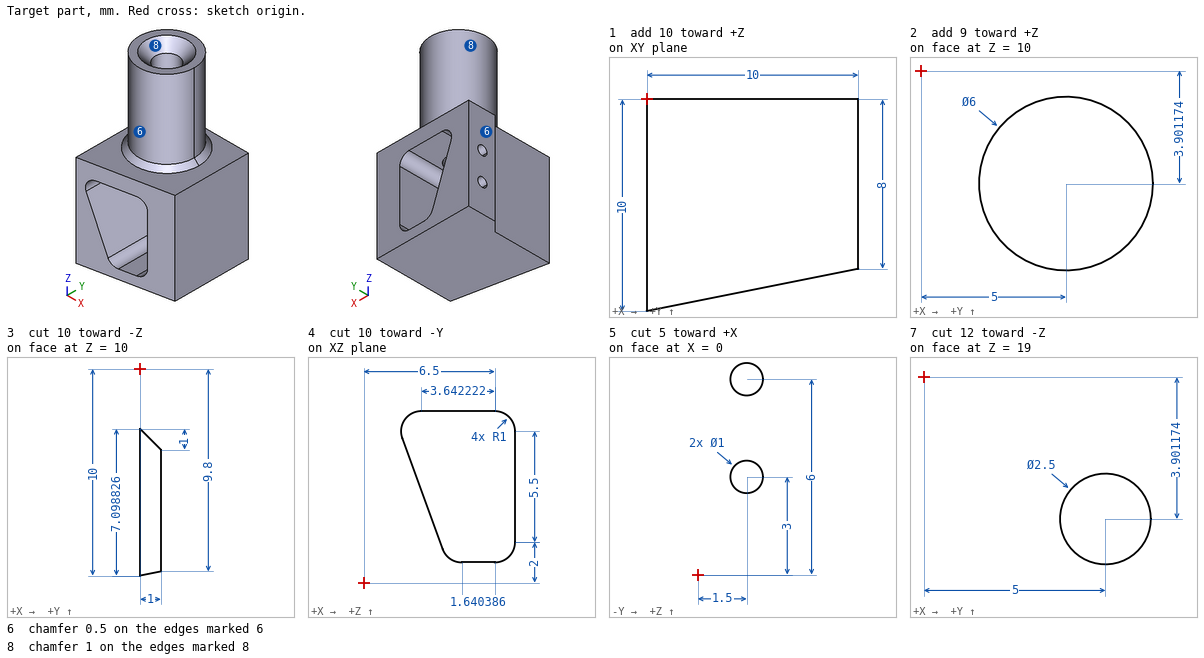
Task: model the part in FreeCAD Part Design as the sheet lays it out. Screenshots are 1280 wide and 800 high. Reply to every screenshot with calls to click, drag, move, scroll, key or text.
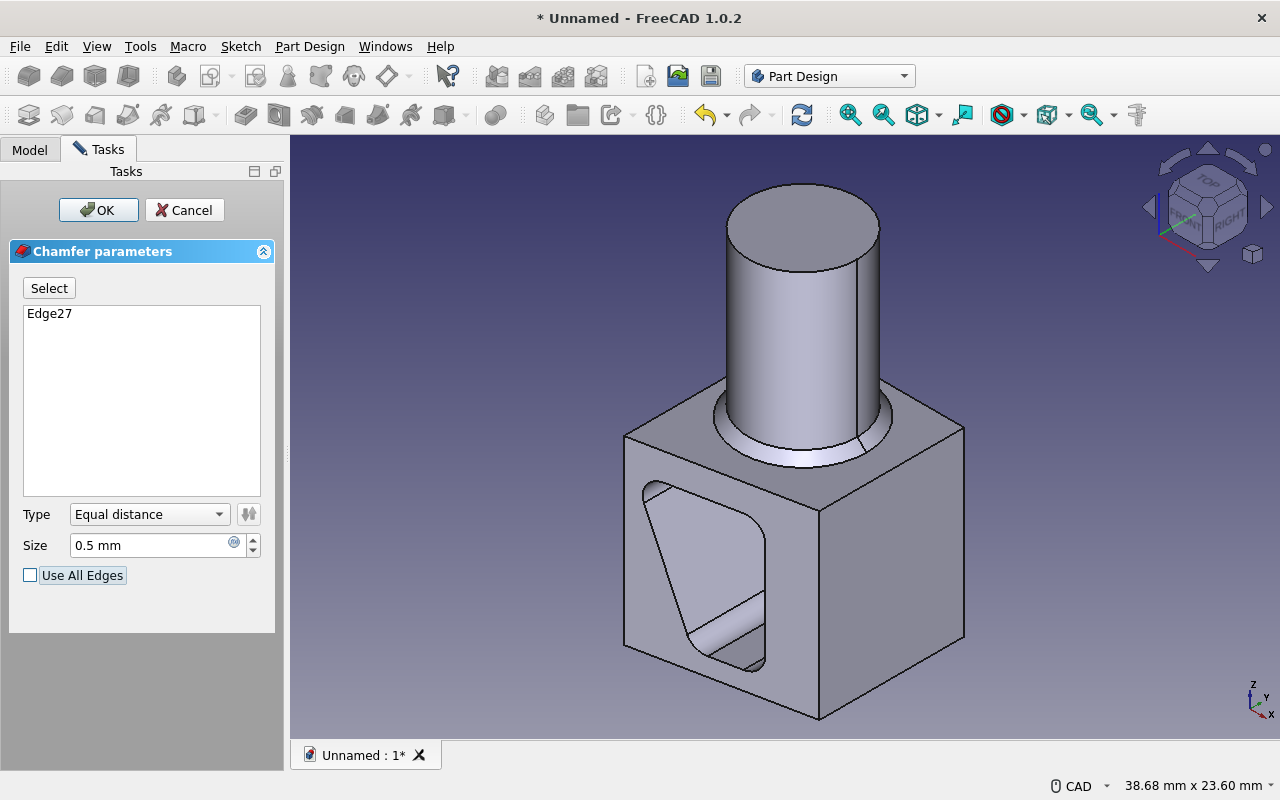
click(99, 210)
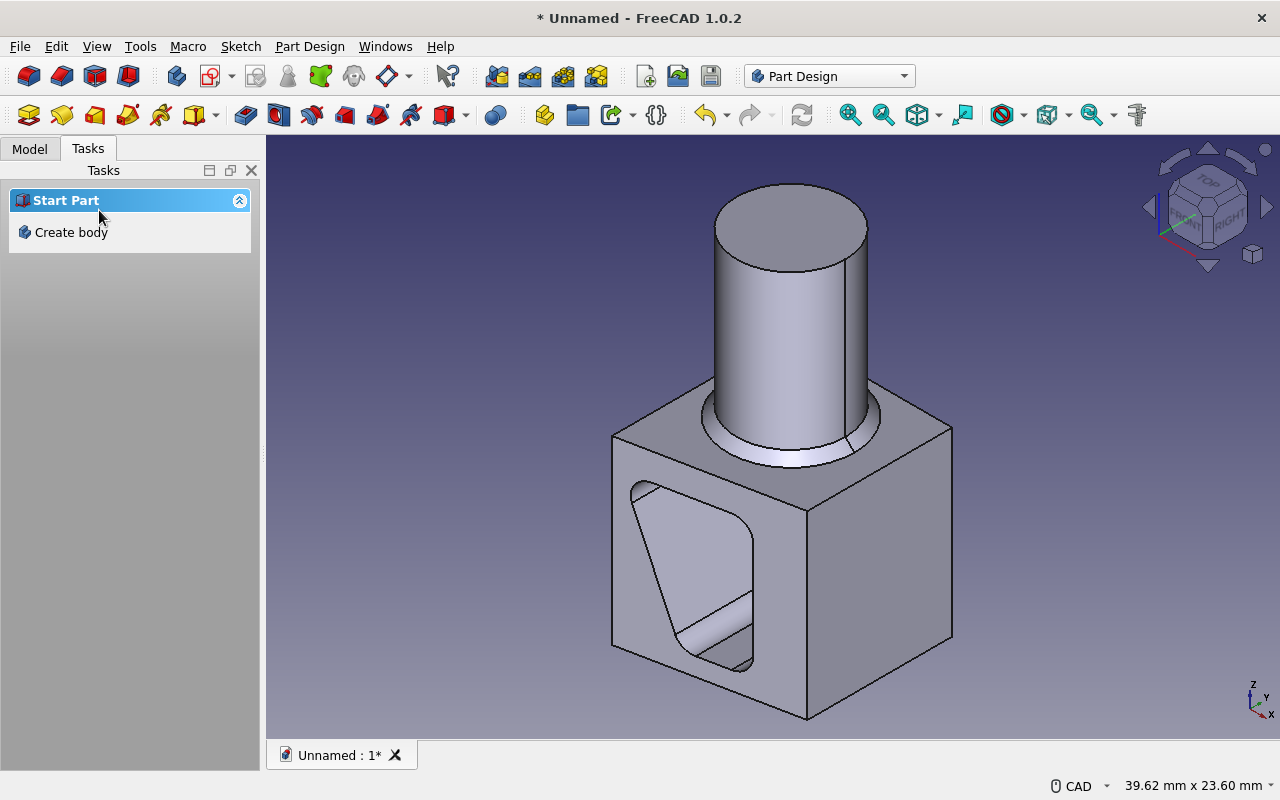
click(851, 116)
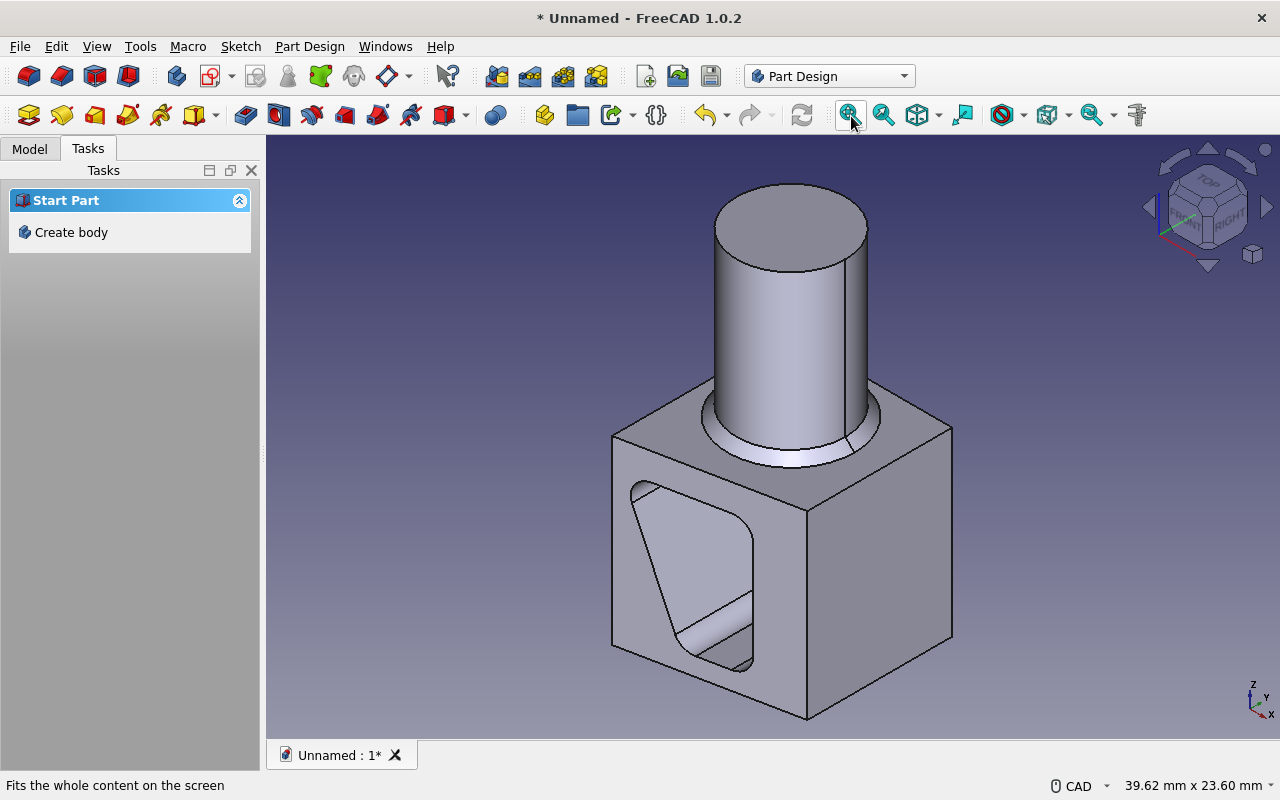
click(791, 227)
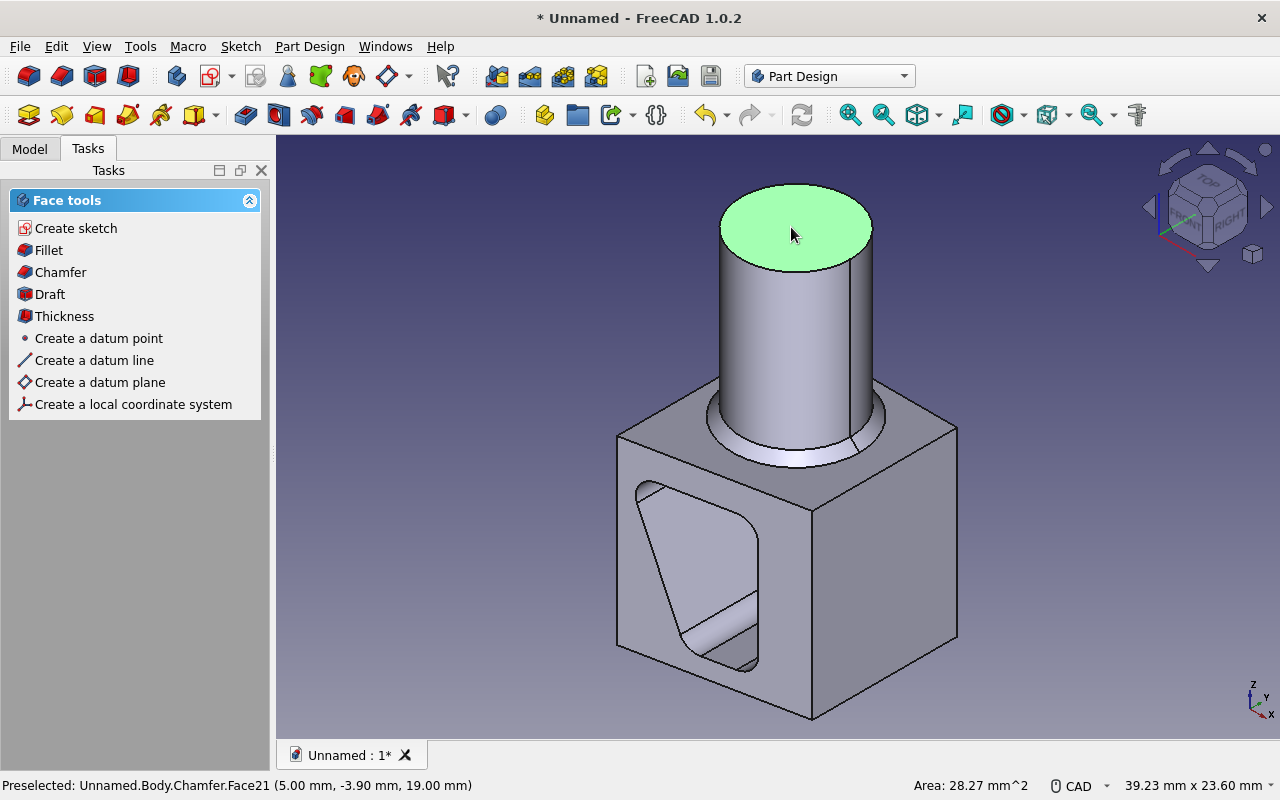
click(210, 76)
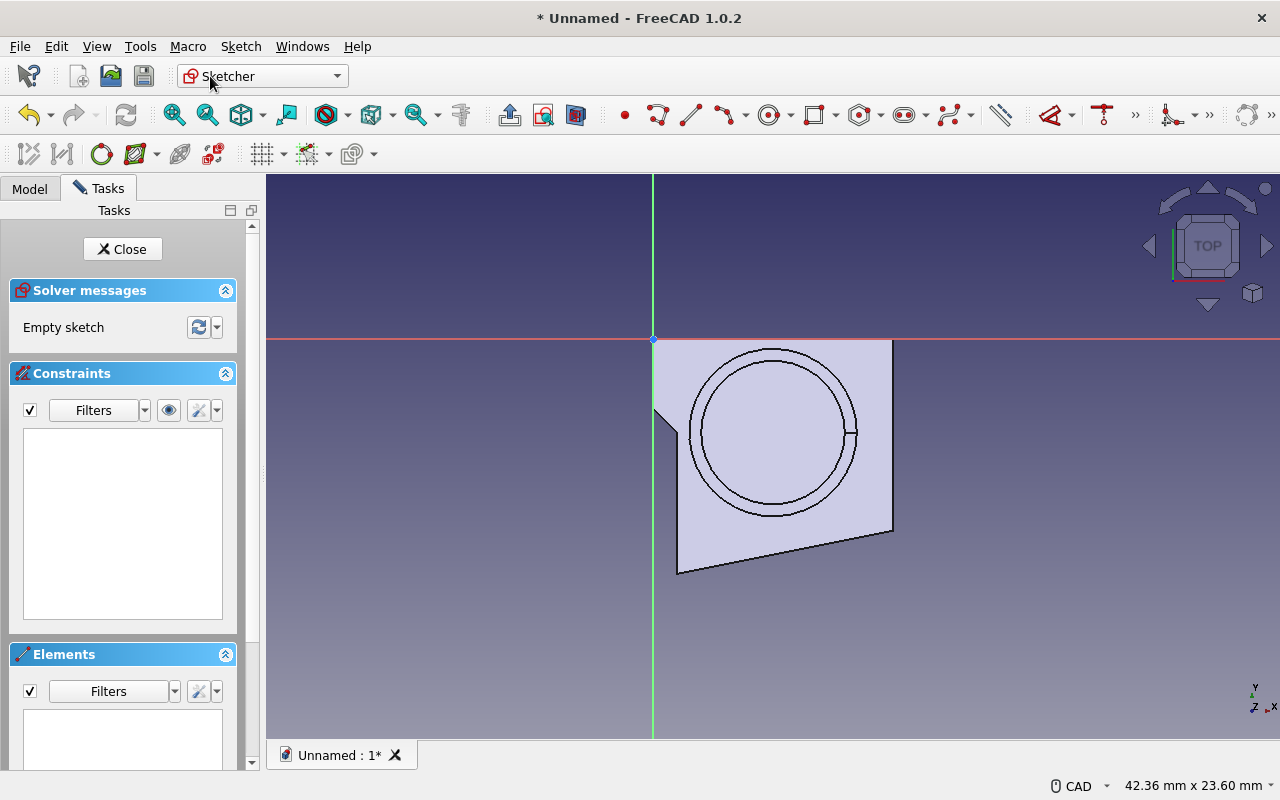
scroll(742, 368, up, 5)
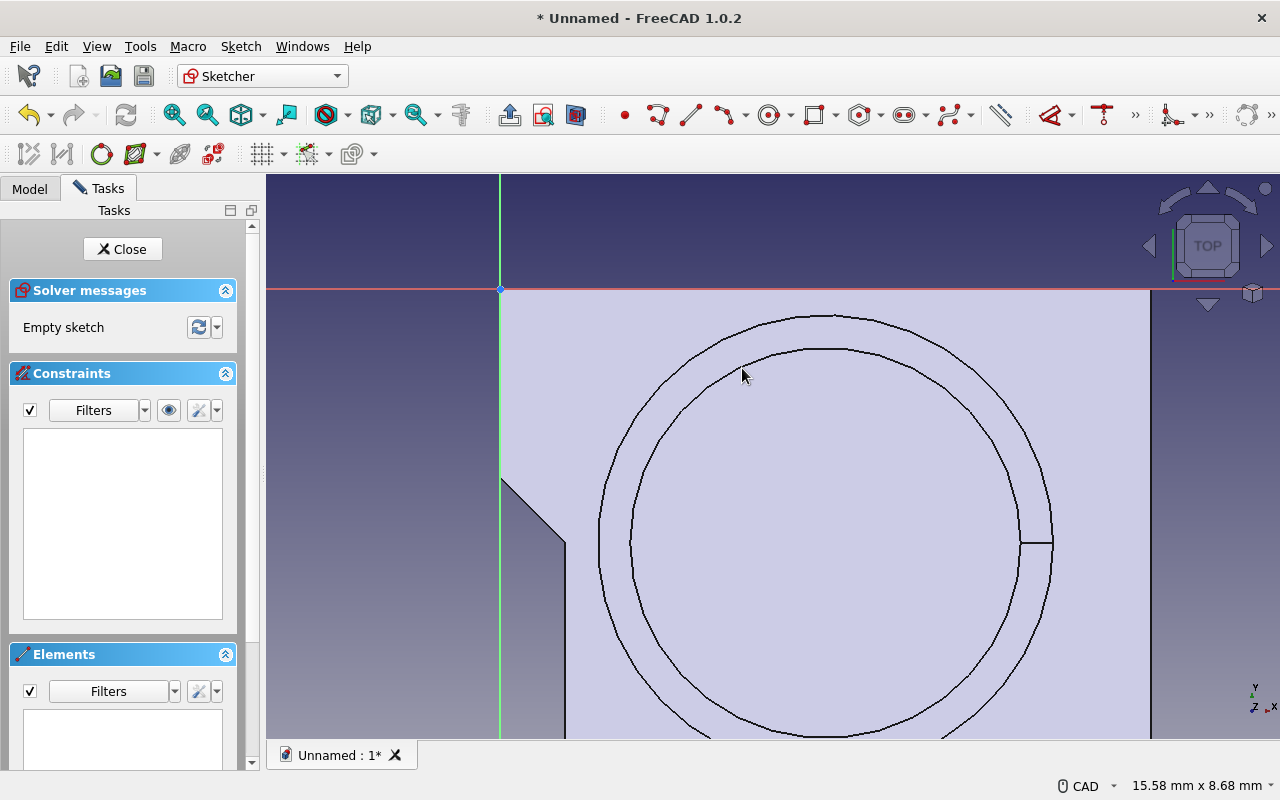
key(g)
key(c)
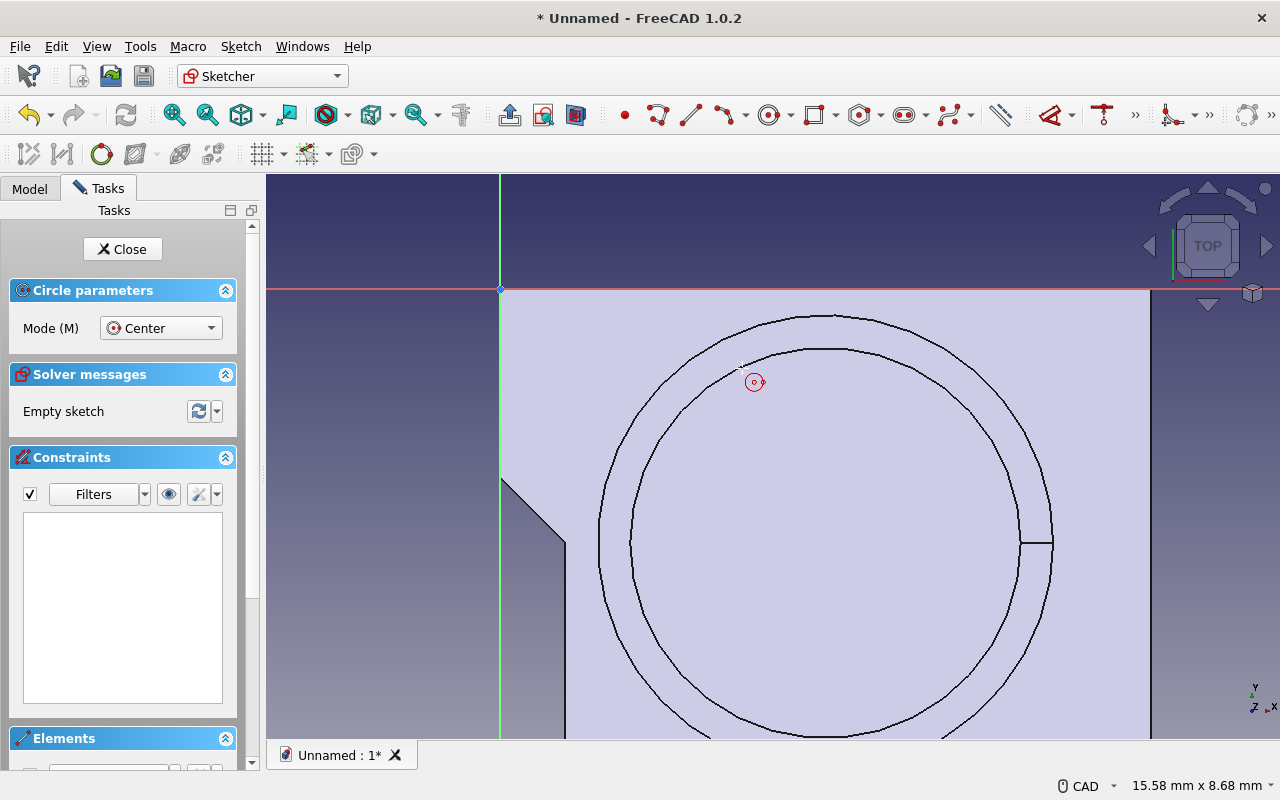
click(825, 543)
click(883, 485)
key(Escape)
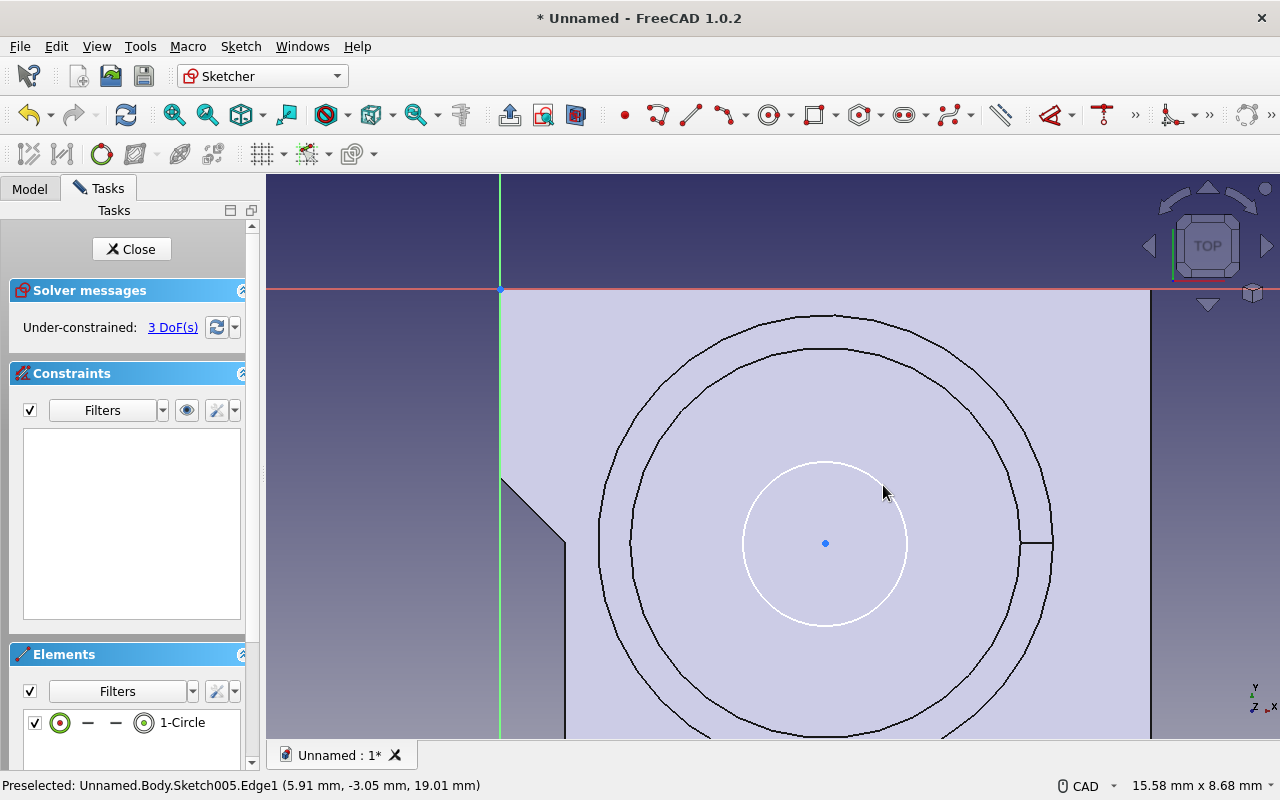
key(d)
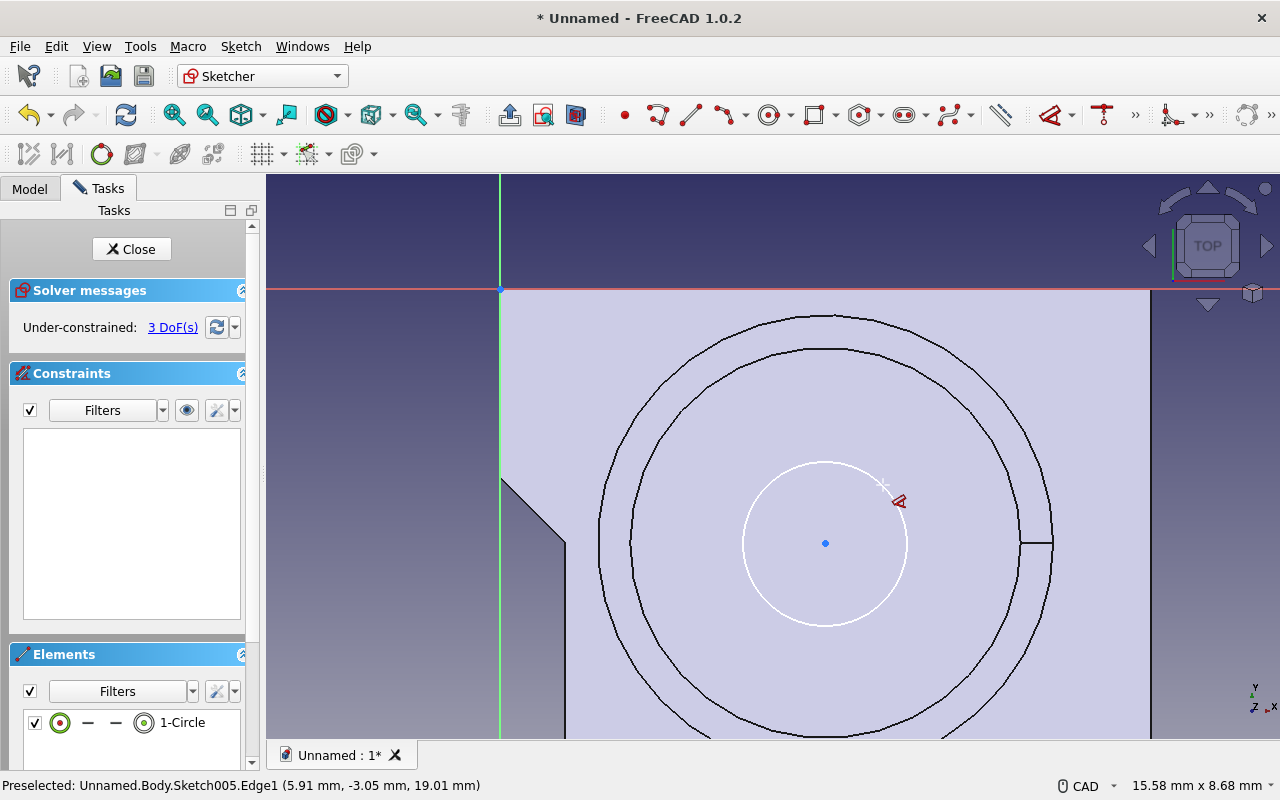
click(883, 486)
click(906, 463)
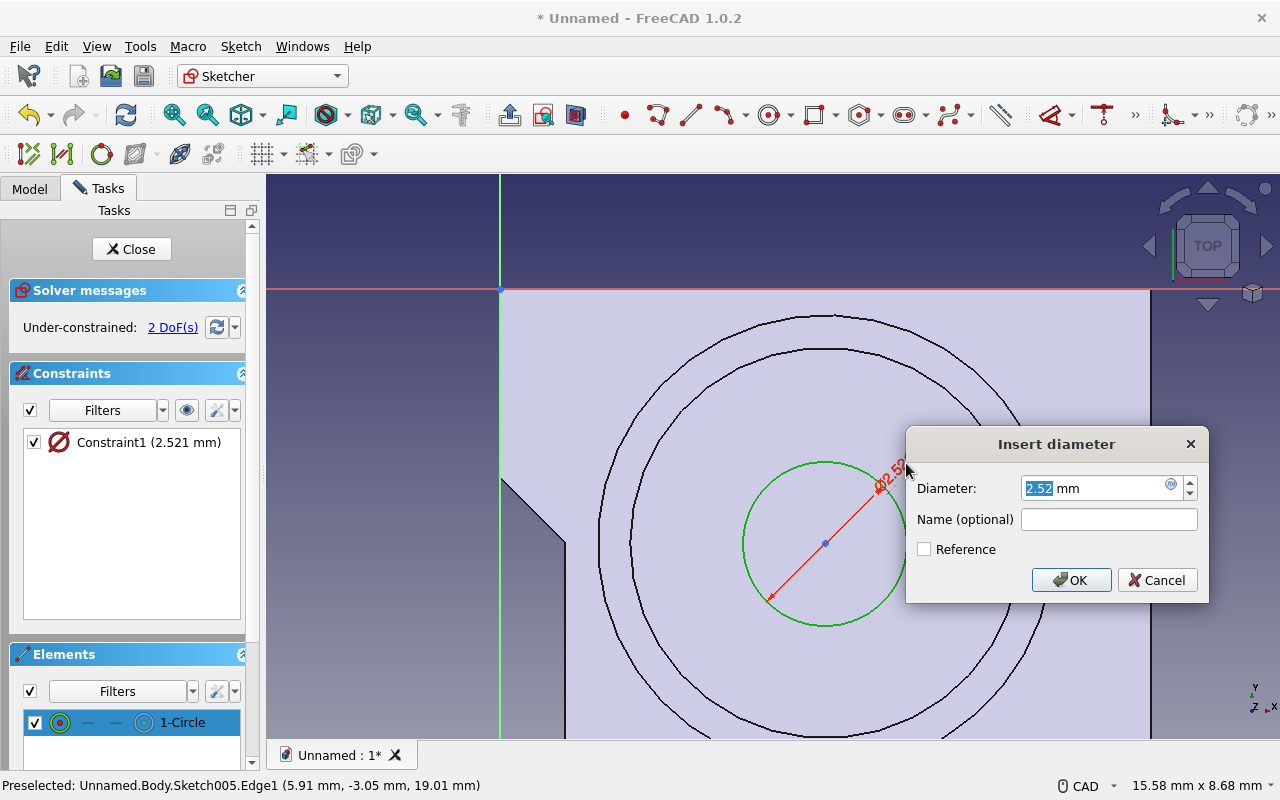
text(2.5)
key(Return)